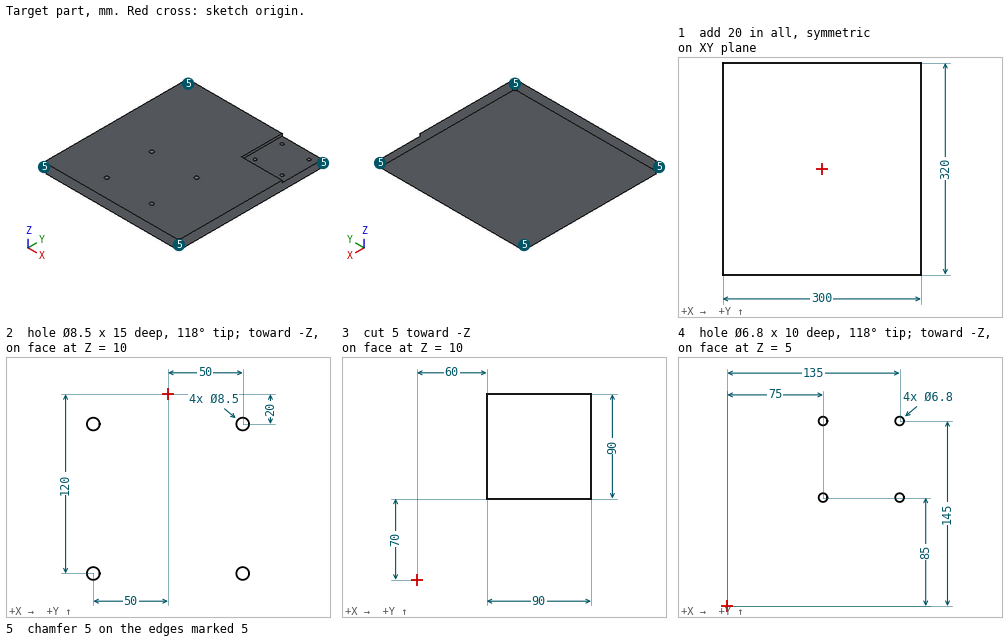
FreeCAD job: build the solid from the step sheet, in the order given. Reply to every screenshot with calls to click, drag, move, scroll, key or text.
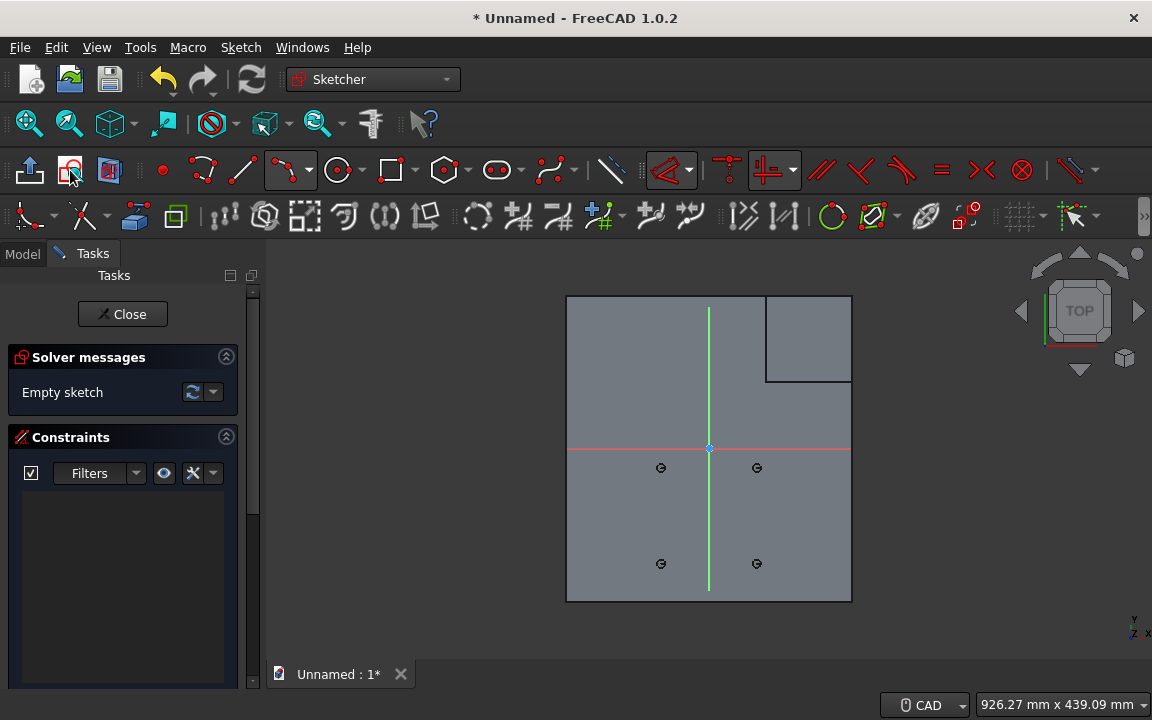
scroll(939, 292, up, 3)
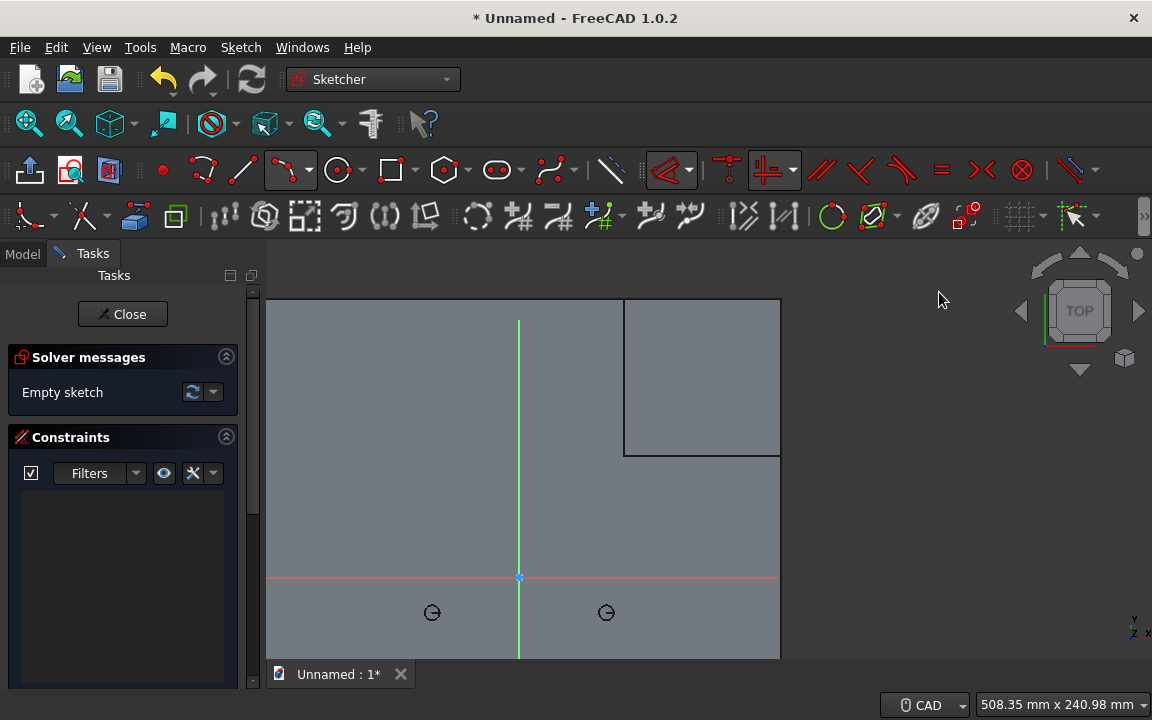
key(g)
key(c)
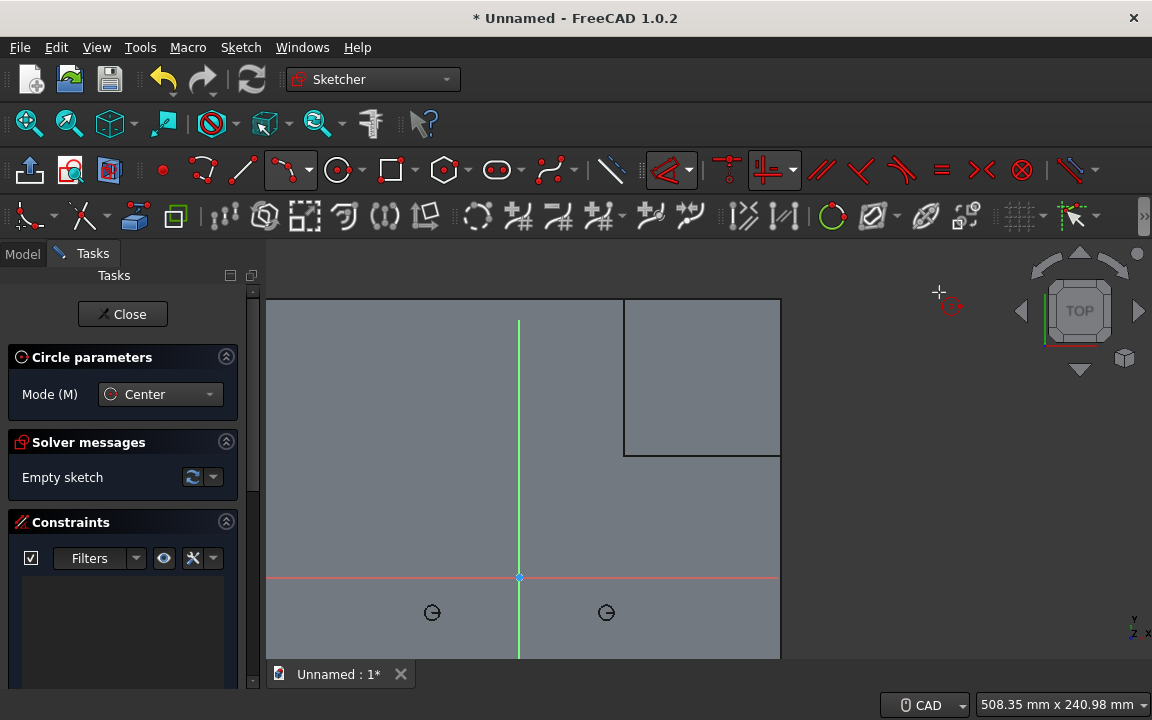
scroll(755, 325, up, 7)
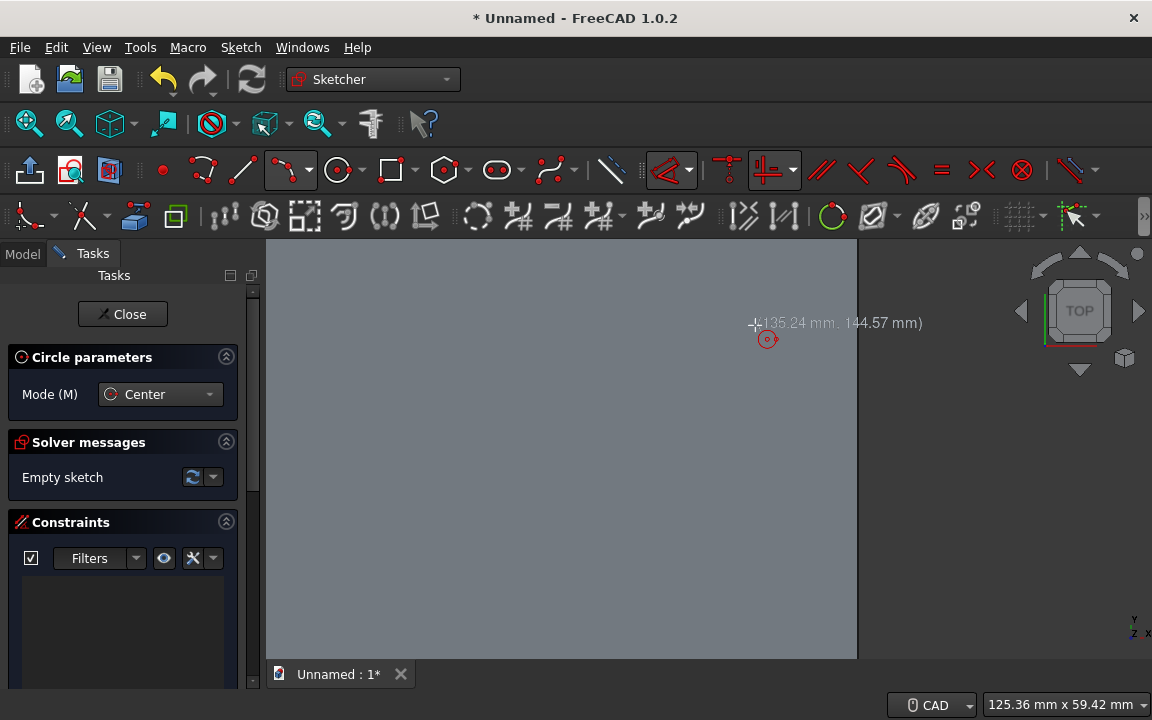
scroll(756, 326, down, 7)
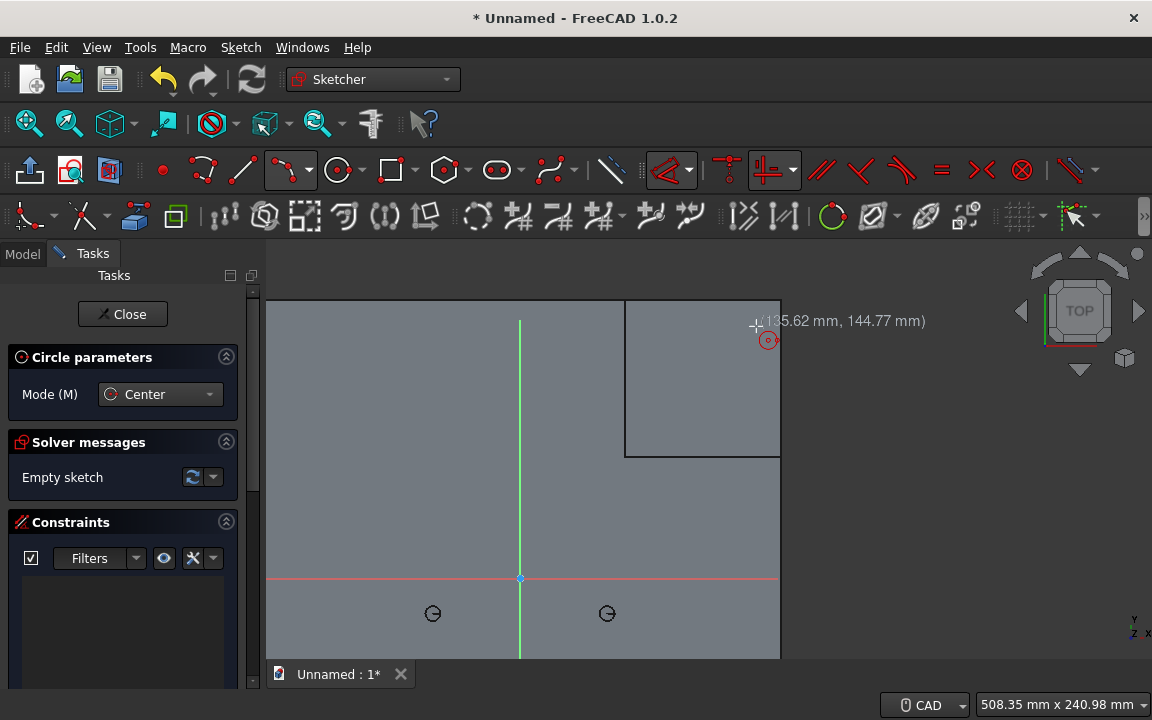
click(755, 326)
move(760, 322)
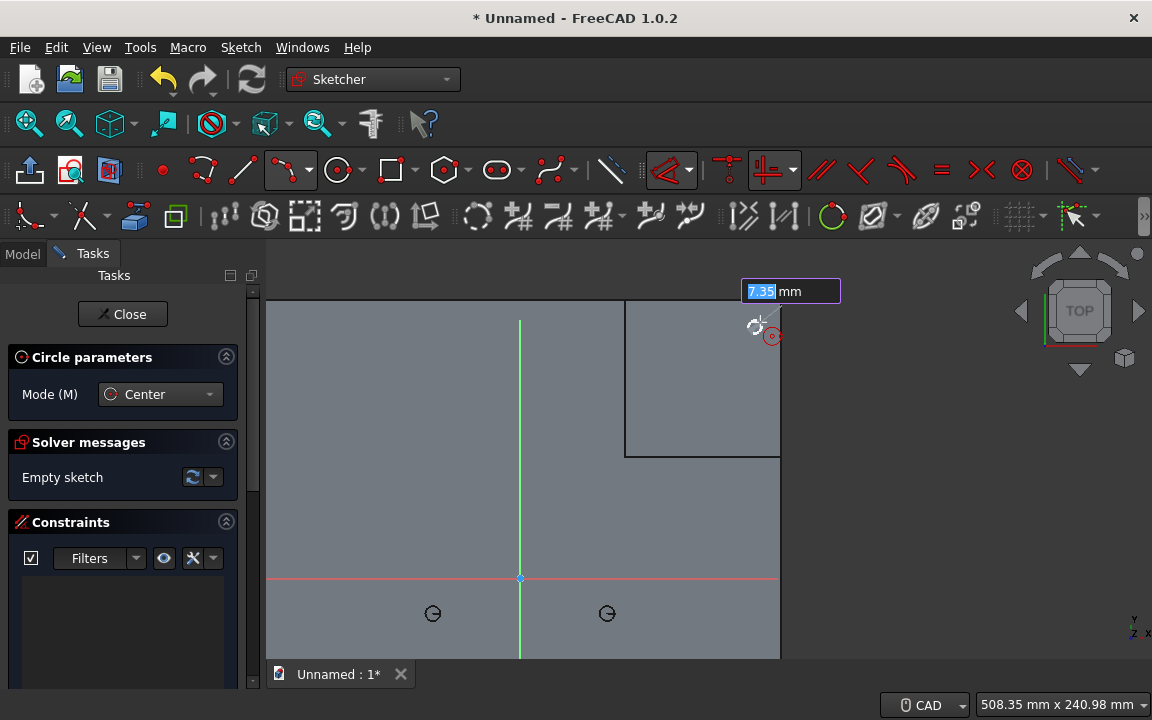
text(6.8)
key(Return)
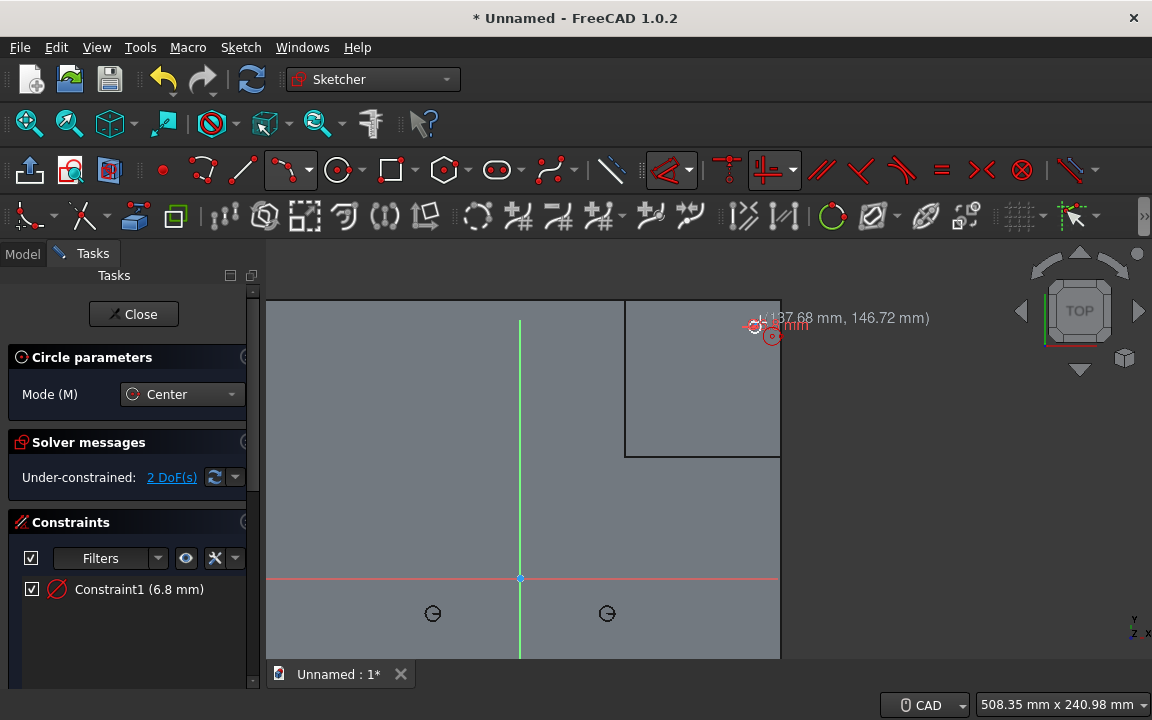
scroll(651, 431, up, 7)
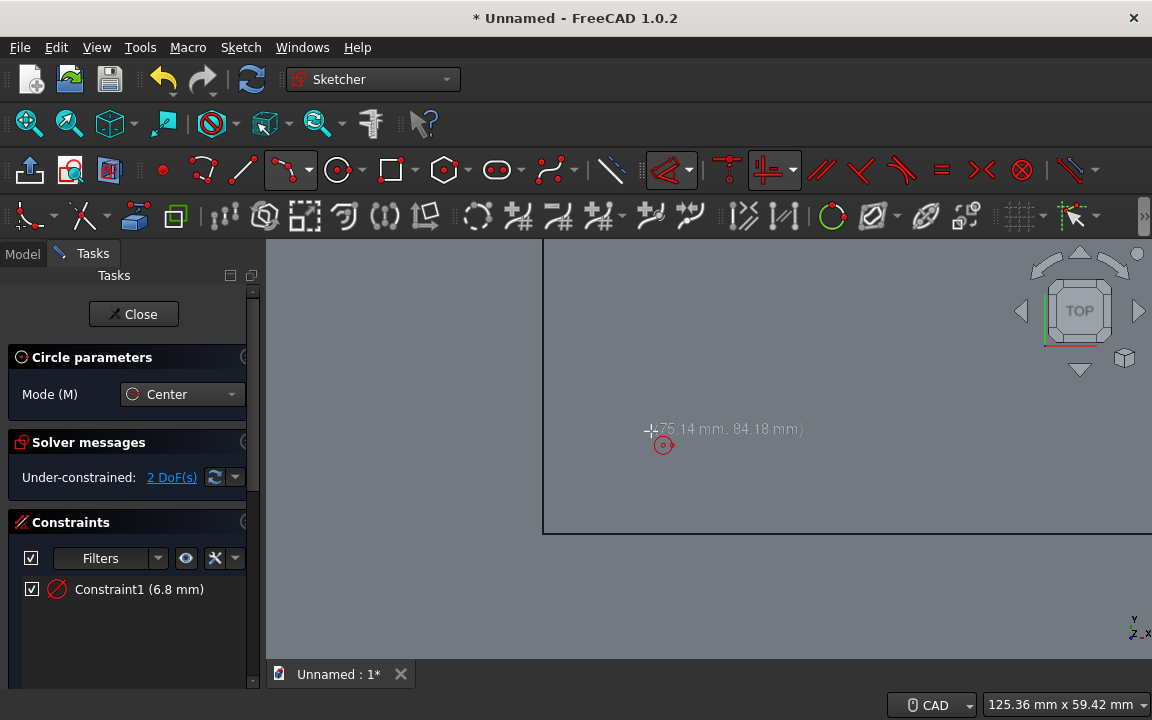
scroll(651, 431, down, 7)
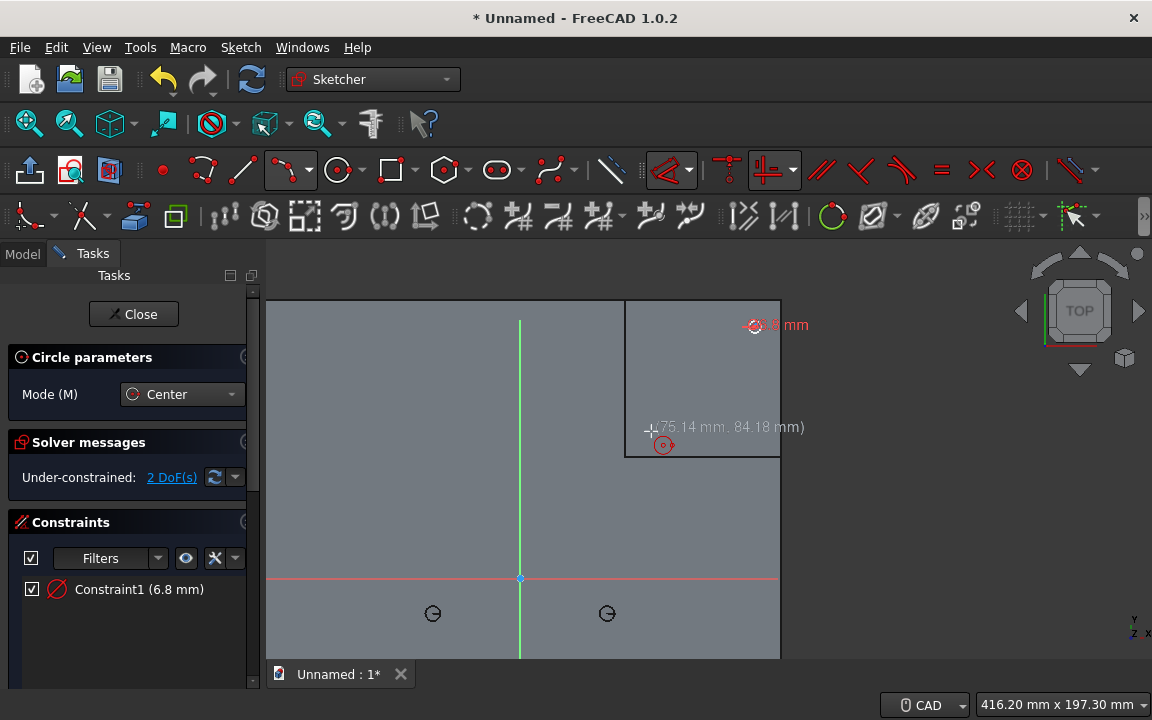
click(651, 431)
move(655, 426)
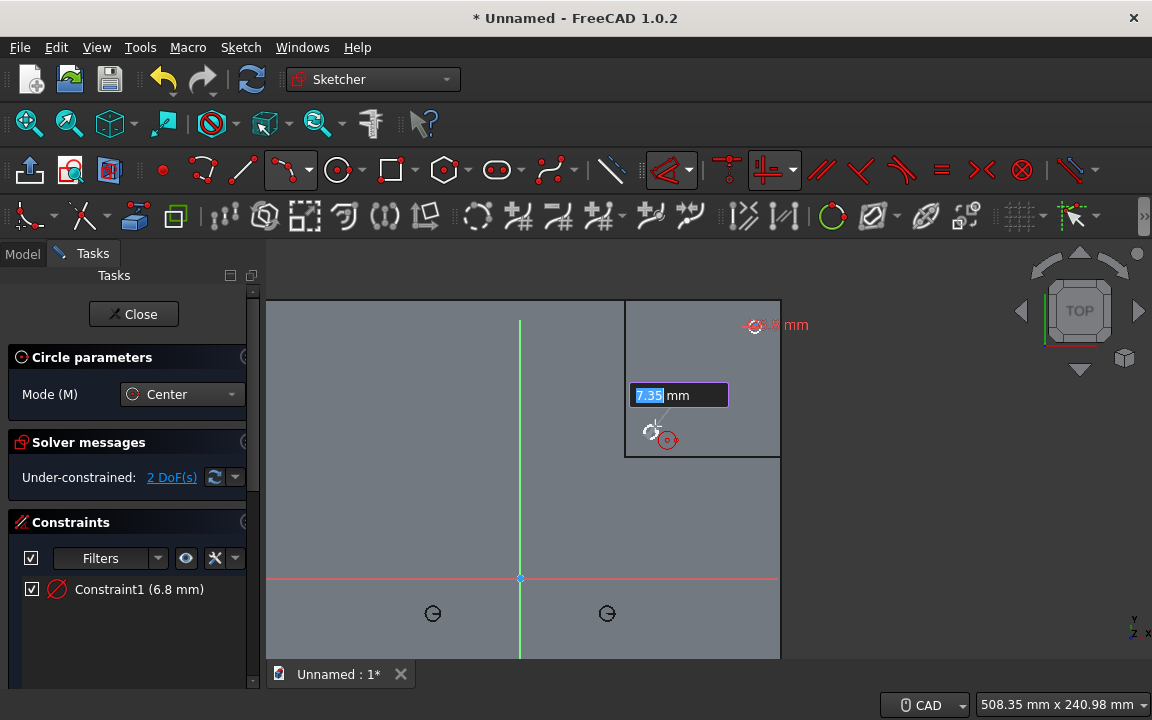
text(6.8)
key(Return)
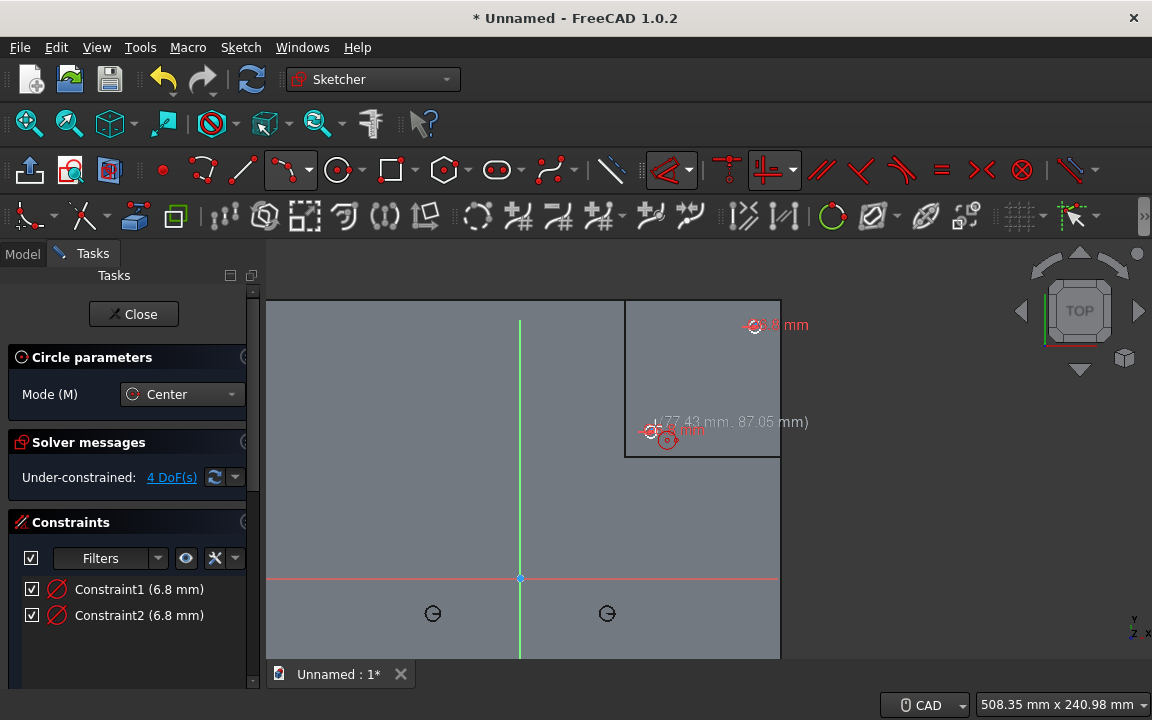
scroll(651, 326, up, 7)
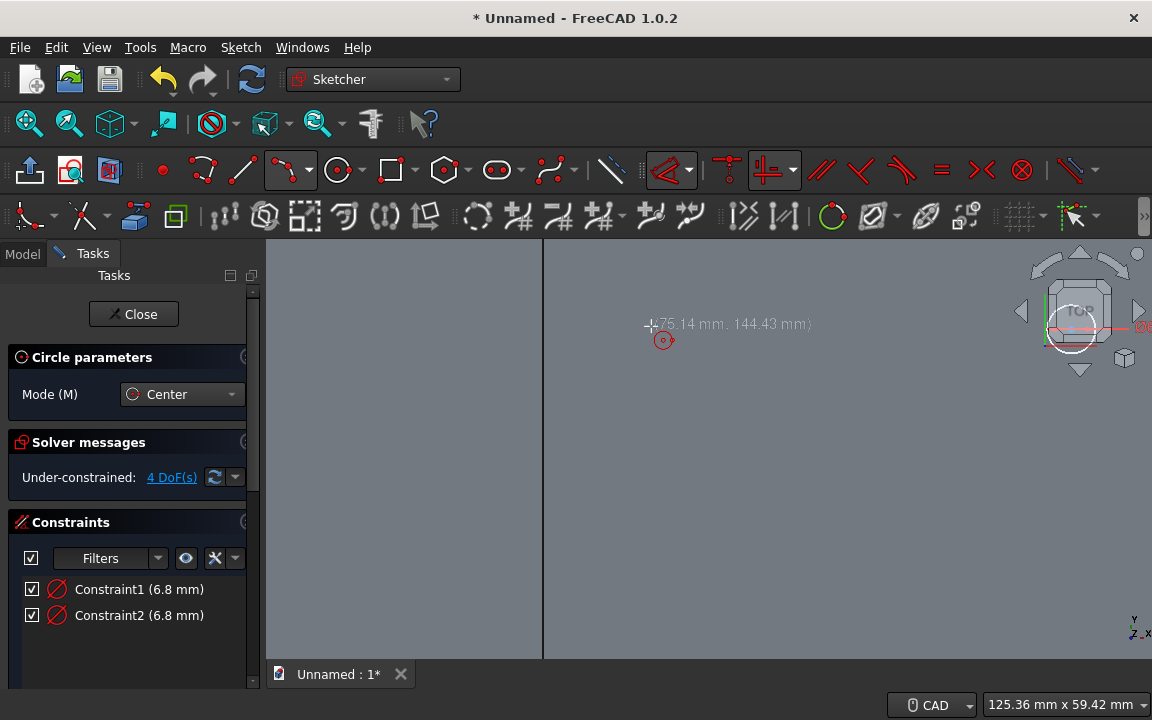
scroll(651, 326, down, 7)